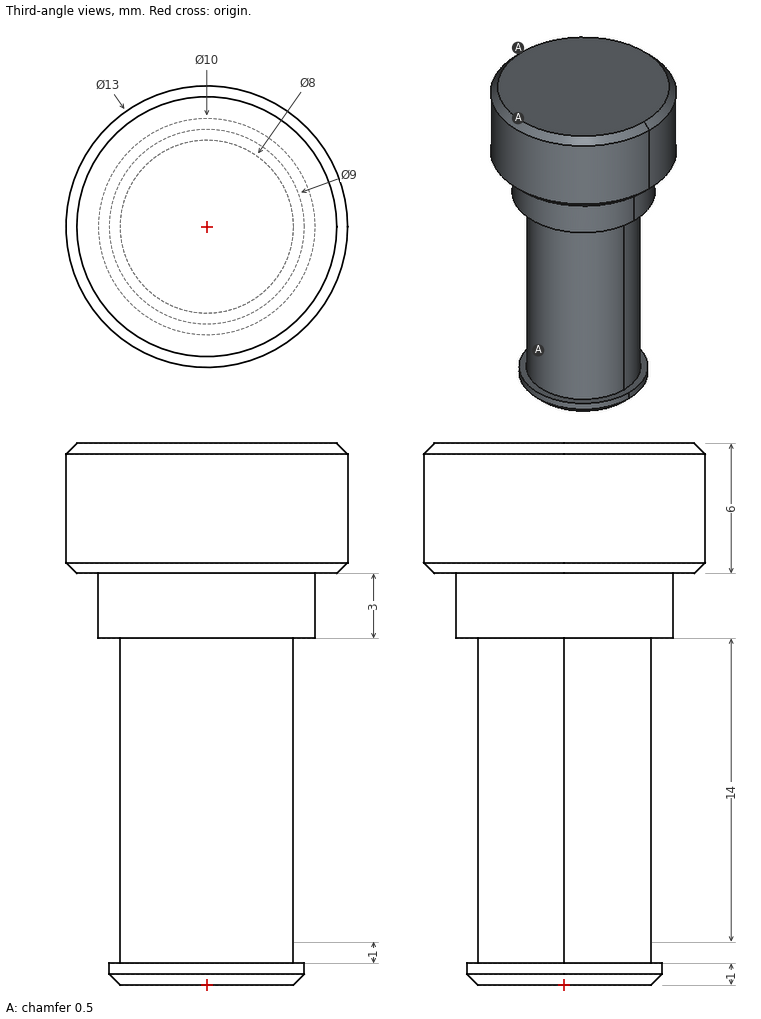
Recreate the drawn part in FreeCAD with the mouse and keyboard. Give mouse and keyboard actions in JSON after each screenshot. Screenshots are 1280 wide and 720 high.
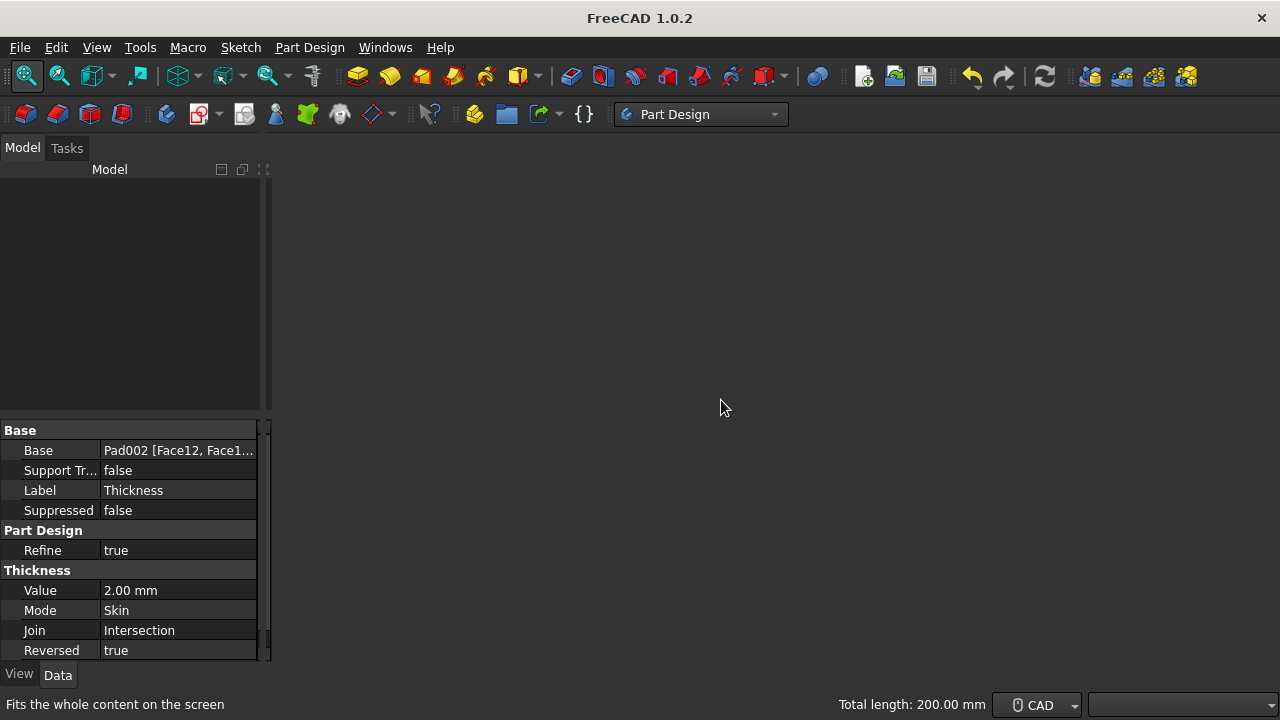
{"action": "left_click", "coordinate": [862, 76]}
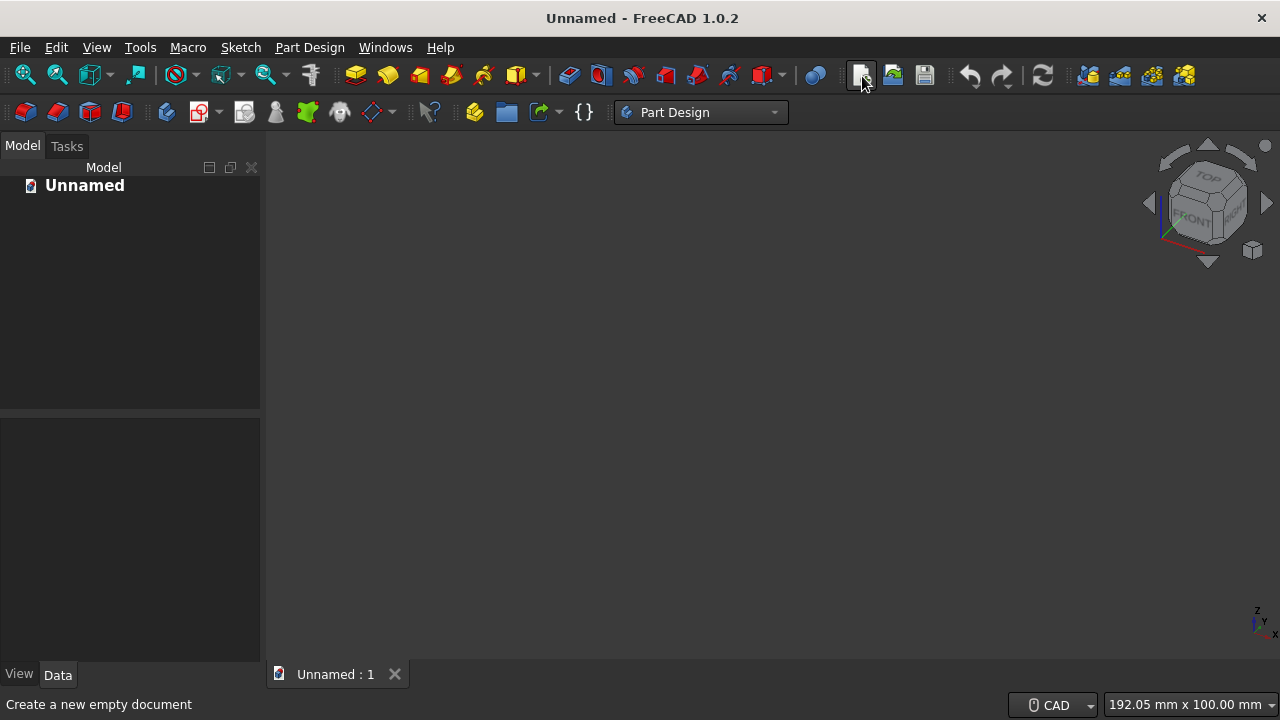
{"action": "left_click", "coordinate": [200, 112]}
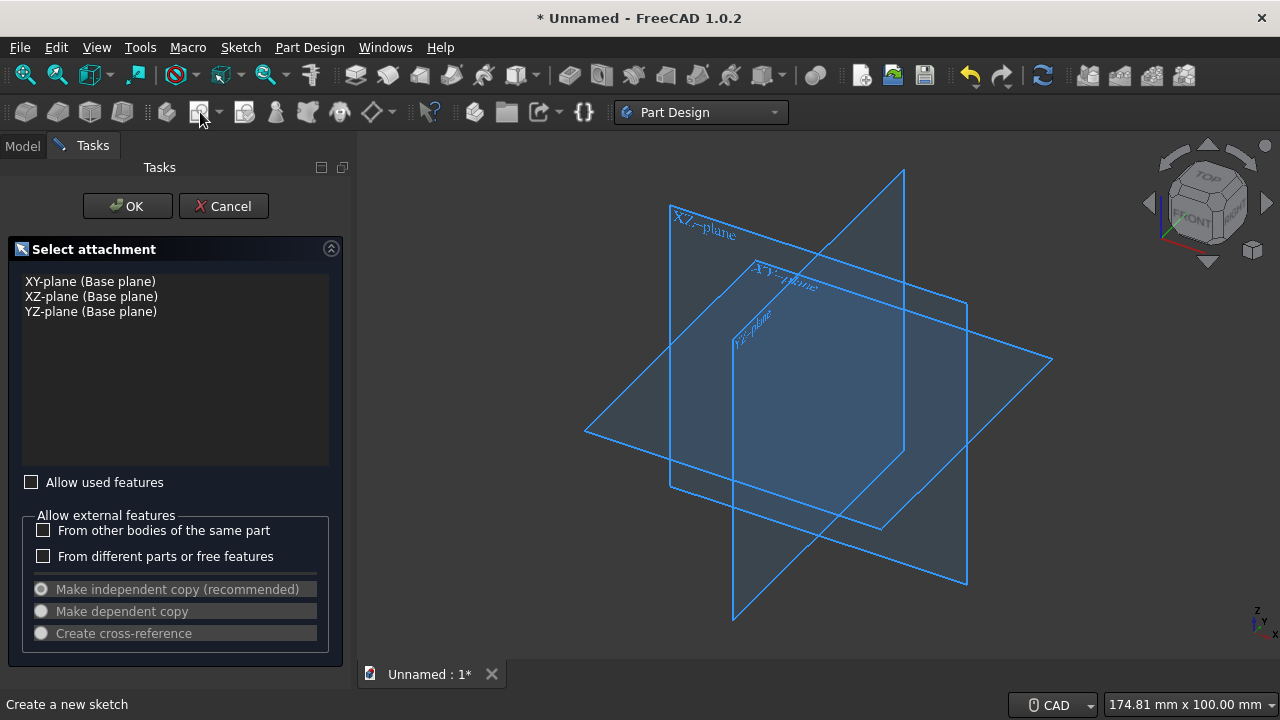
{"action": "left_click", "coordinate": [82, 282]}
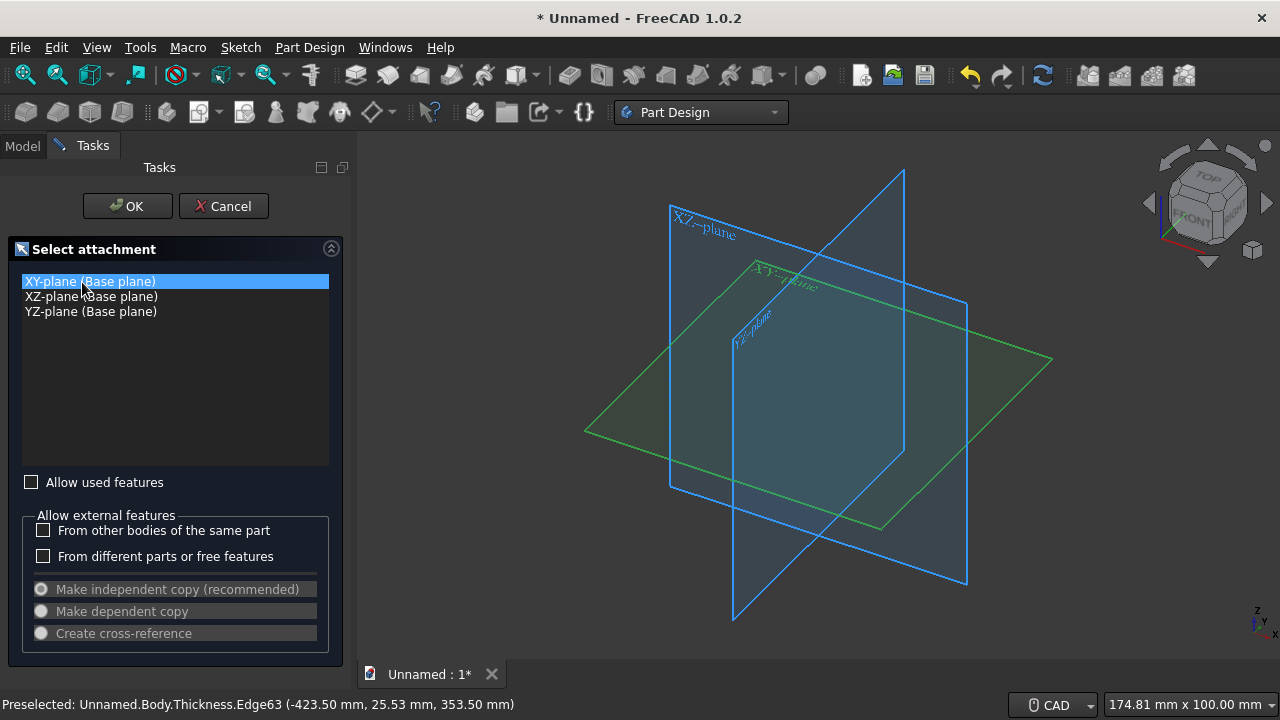
{"action": "left_click", "coordinate": [128, 206]}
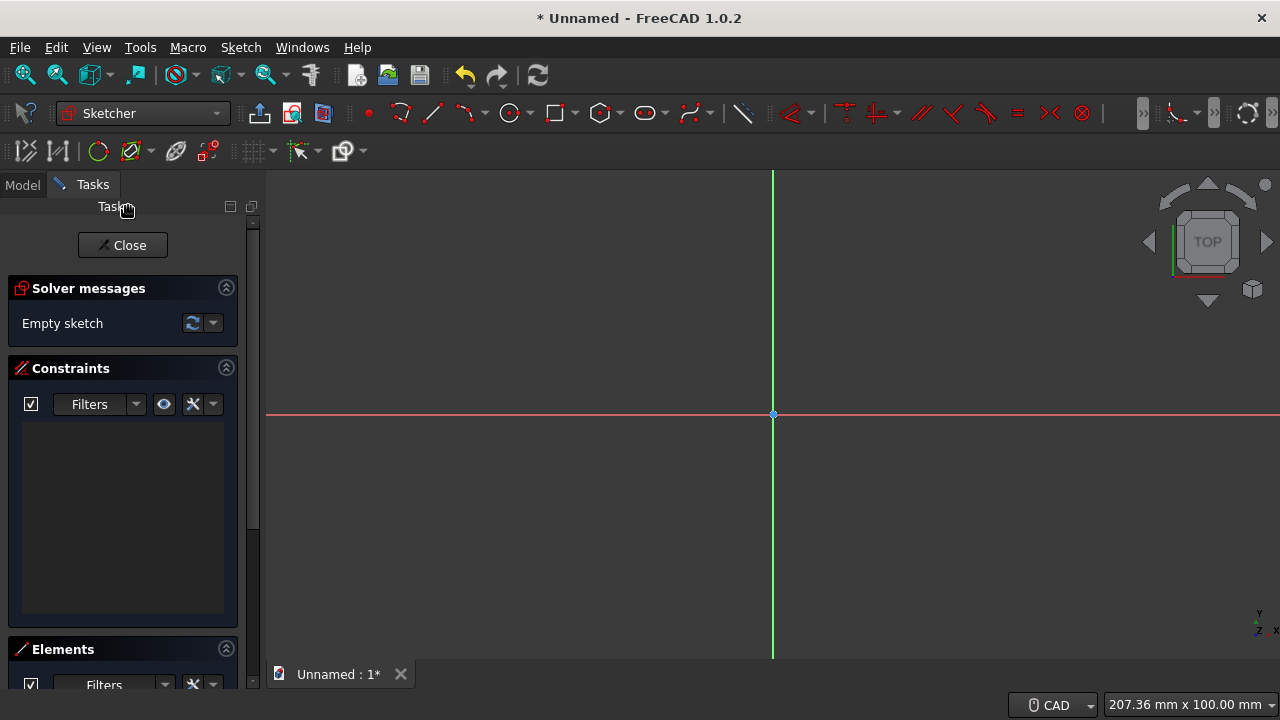
{"action": "scroll", "coordinate": [784, 414], "scroll_direction": "up", "scroll_amount": 10}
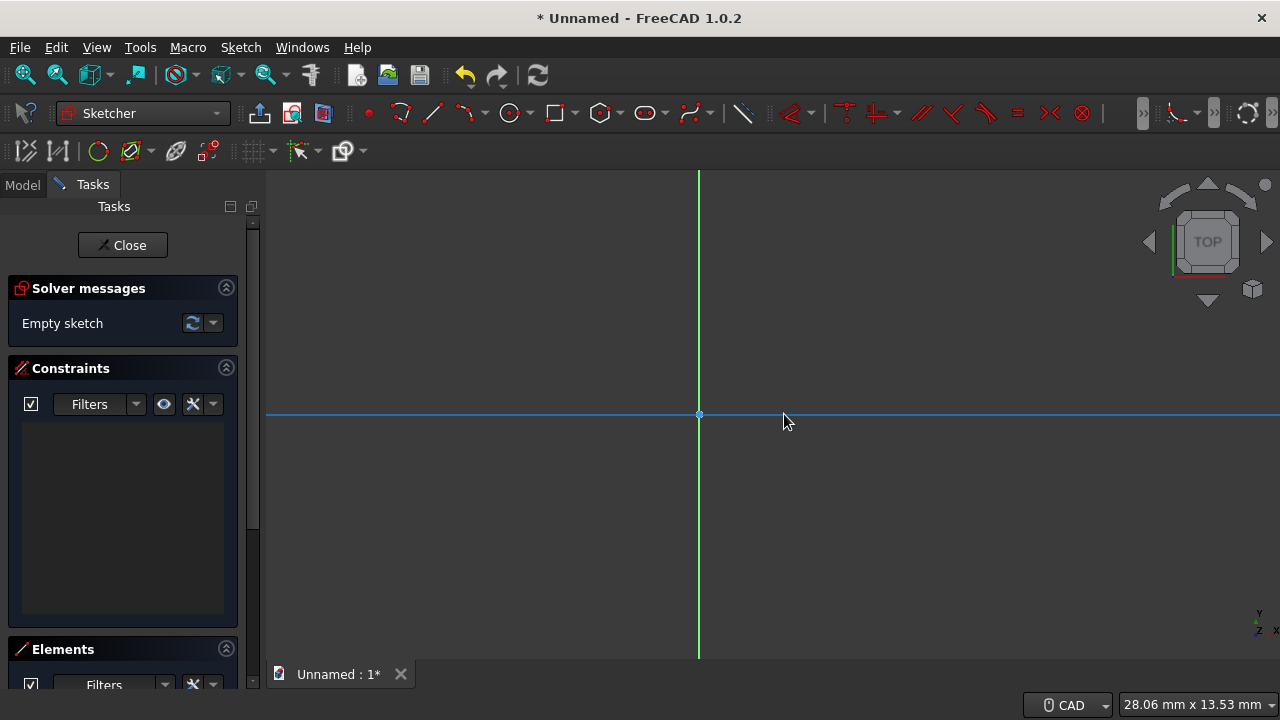
{"action": "left_click", "coordinate": [510, 114]}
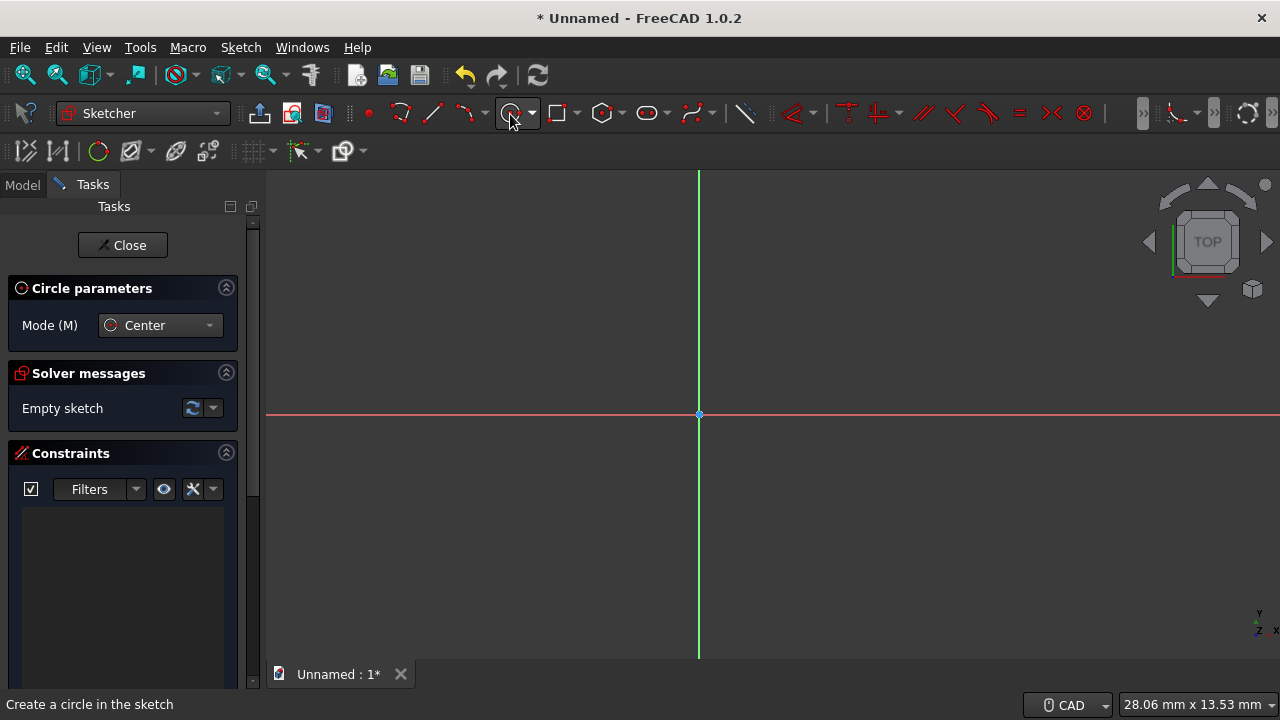
{"action": "left_click", "coordinate": [699, 414]}
{"action": "mouse_move", "coordinate": [814, 300]}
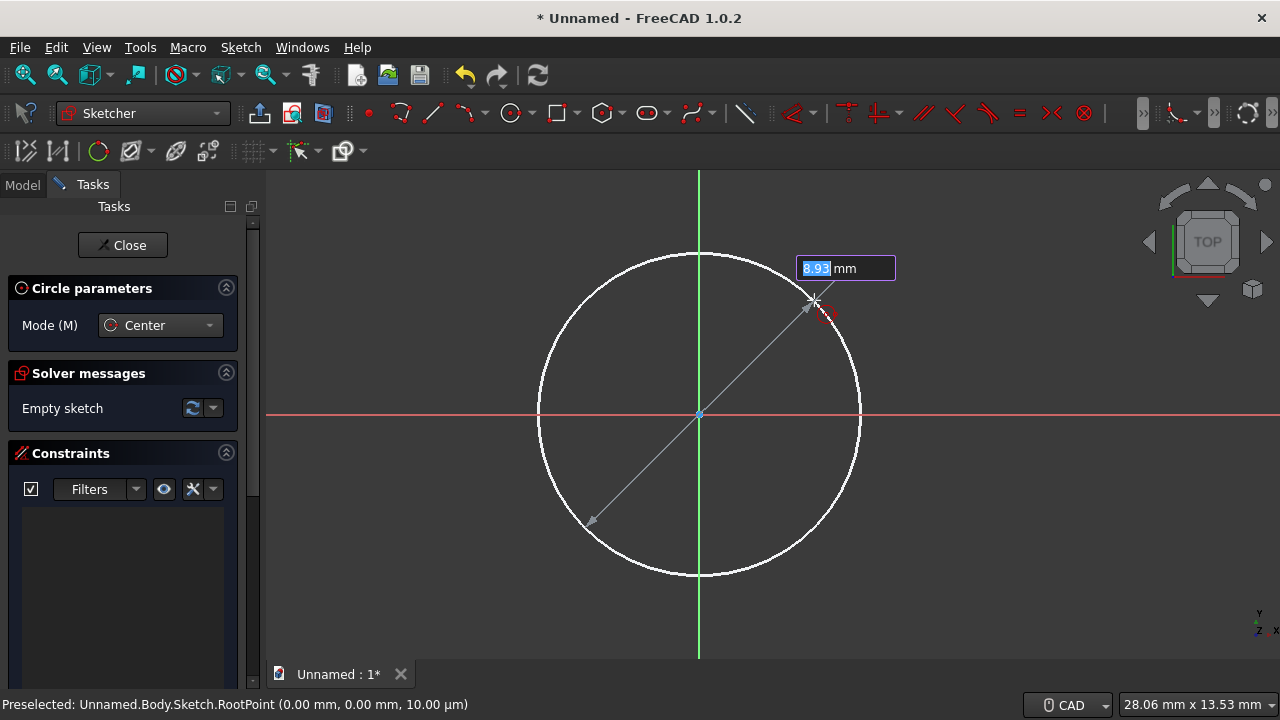
{"action": "type", "text": "9"}
{"action": "key", "text": "Return"}
{"action": "key", "text": "Escape"}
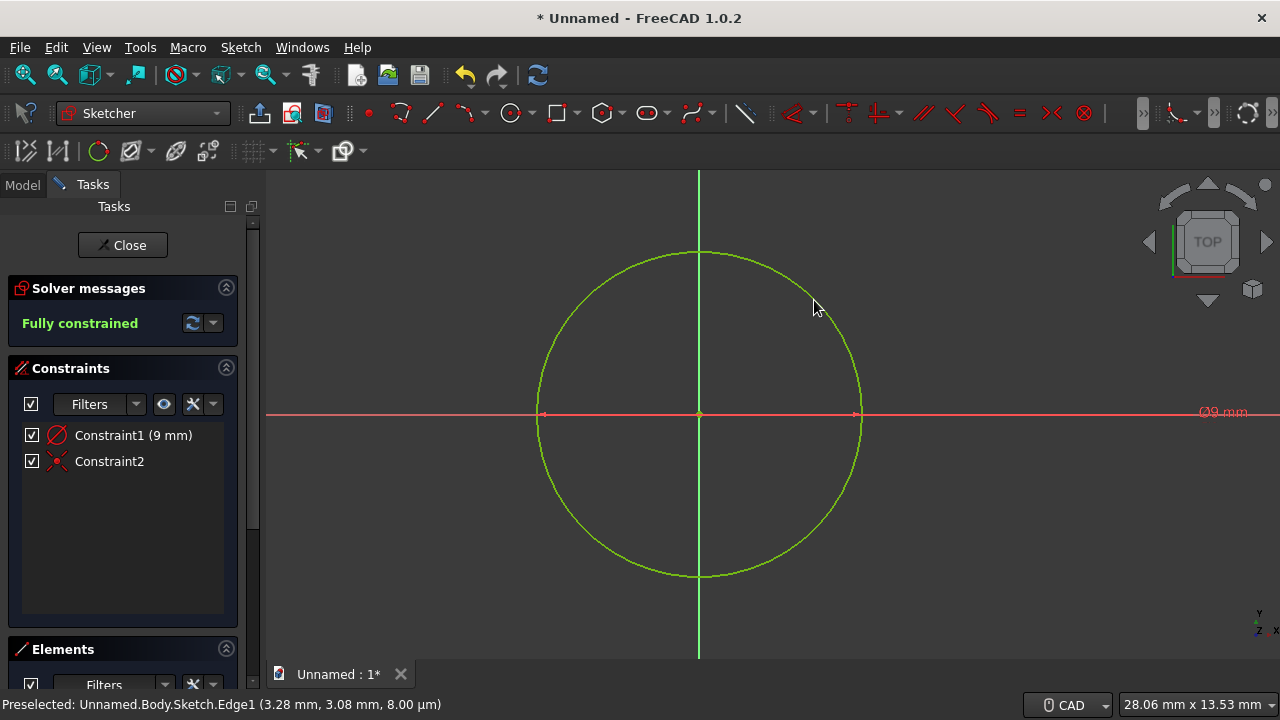
{"action": "left_click", "coordinate": [123, 245]}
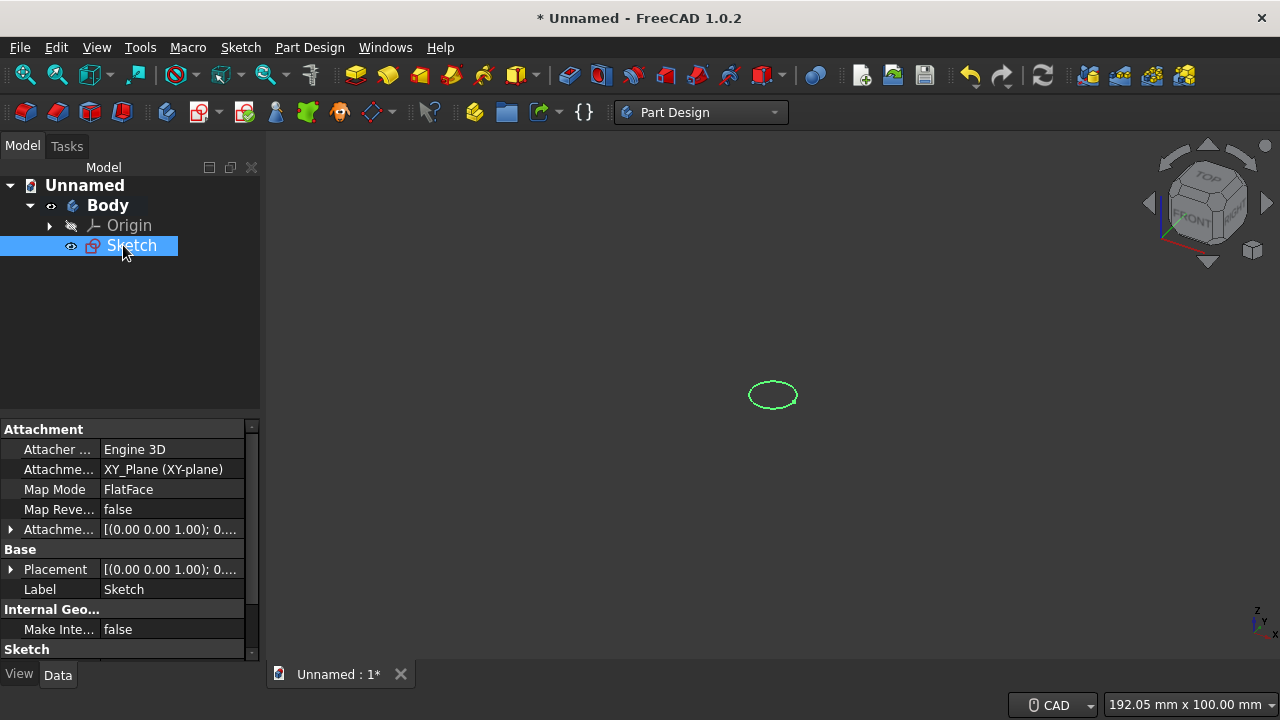
{"action": "left_click", "coordinate": [356, 76]}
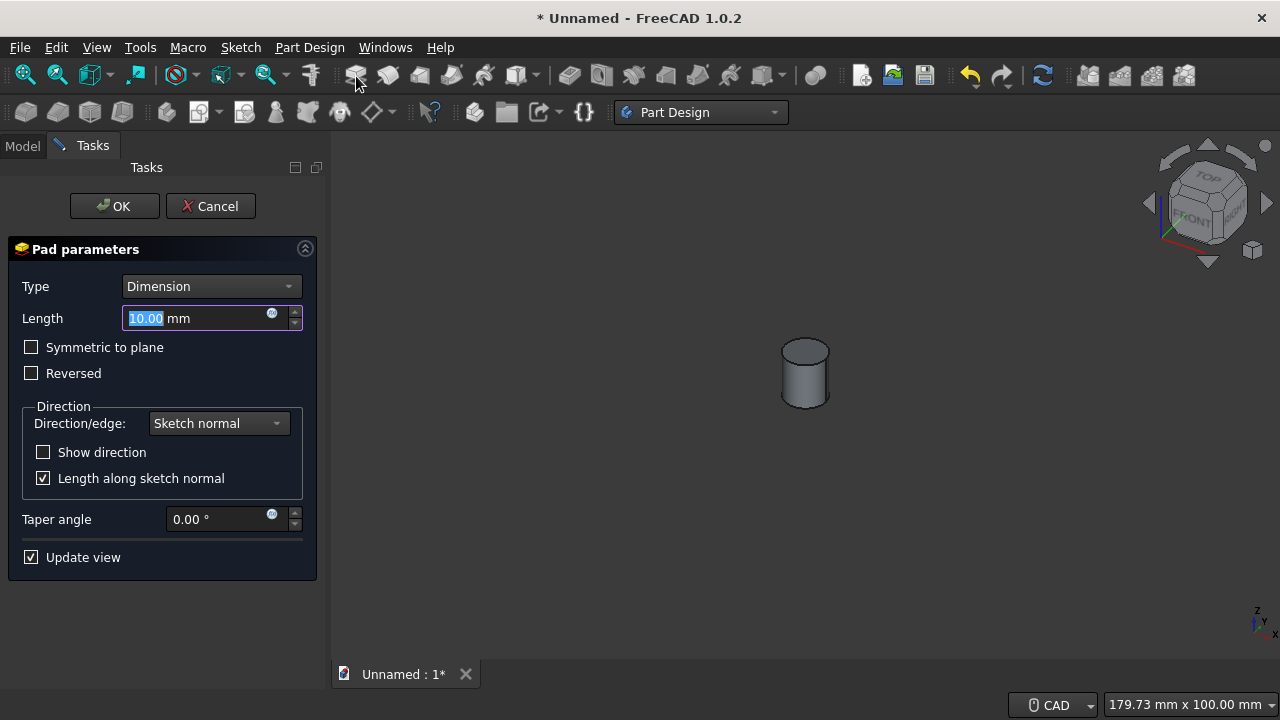
{"action": "type", "text": "1"}
{"action": "key", "text": "Tab"}